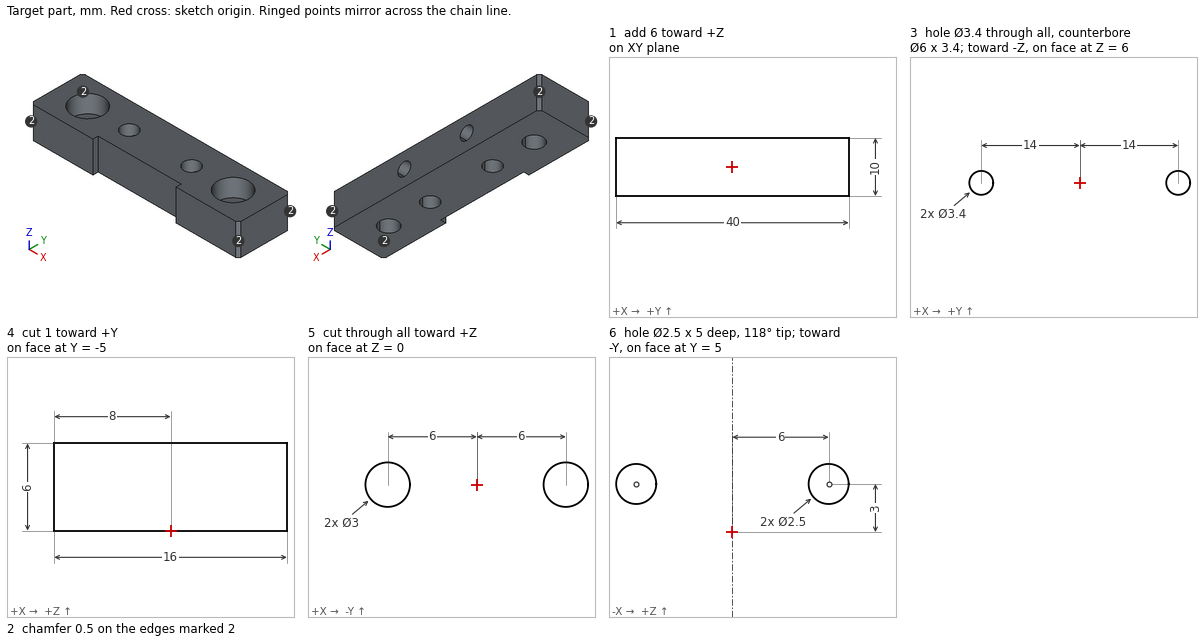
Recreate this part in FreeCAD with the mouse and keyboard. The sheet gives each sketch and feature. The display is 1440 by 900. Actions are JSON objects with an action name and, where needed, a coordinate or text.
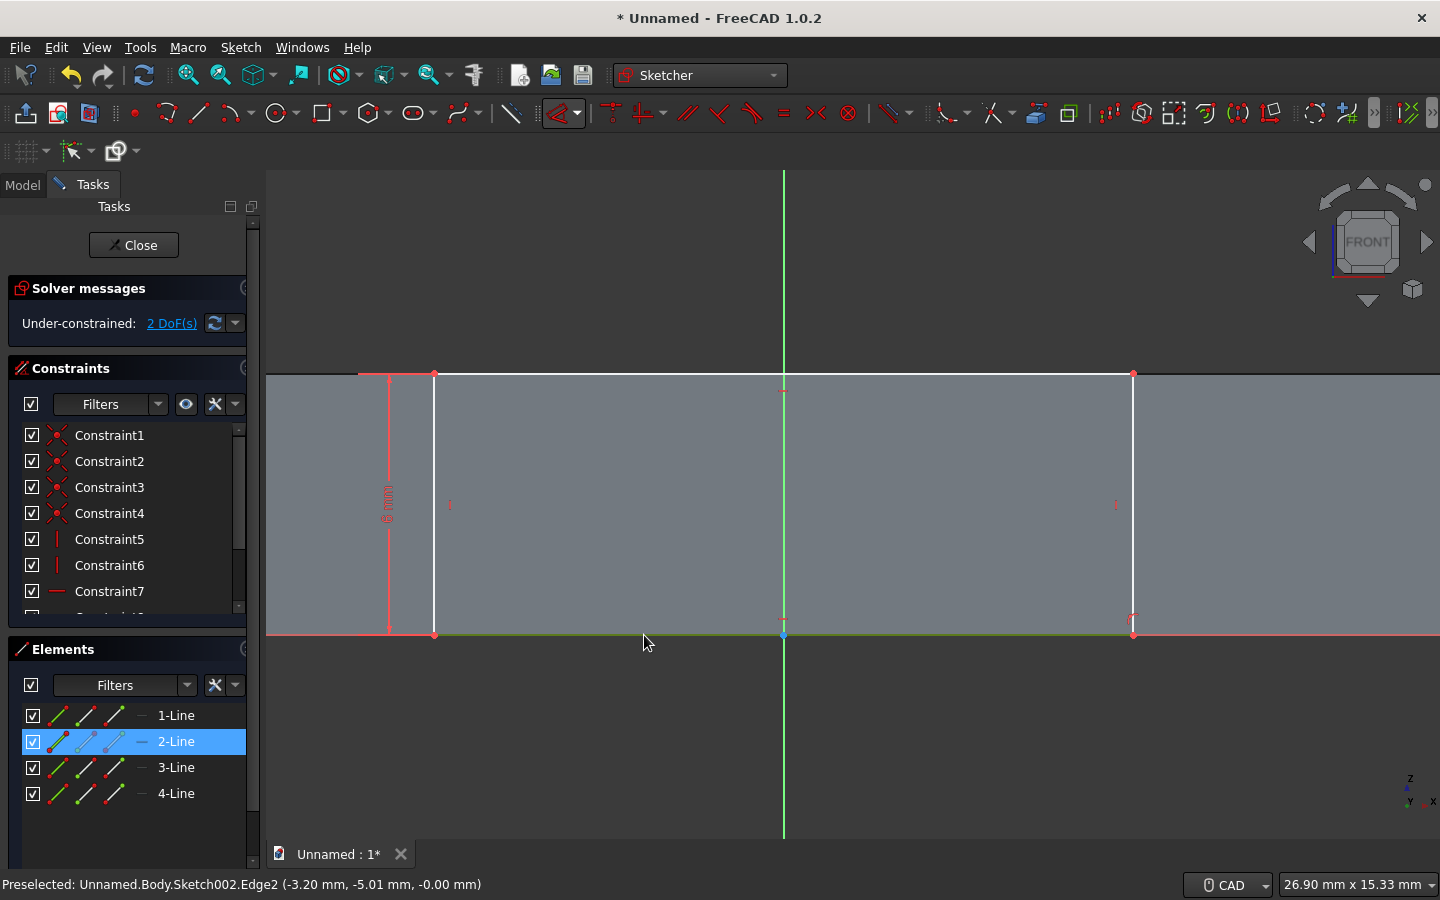
{"action": "left_click", "coordinate": [580, 114]}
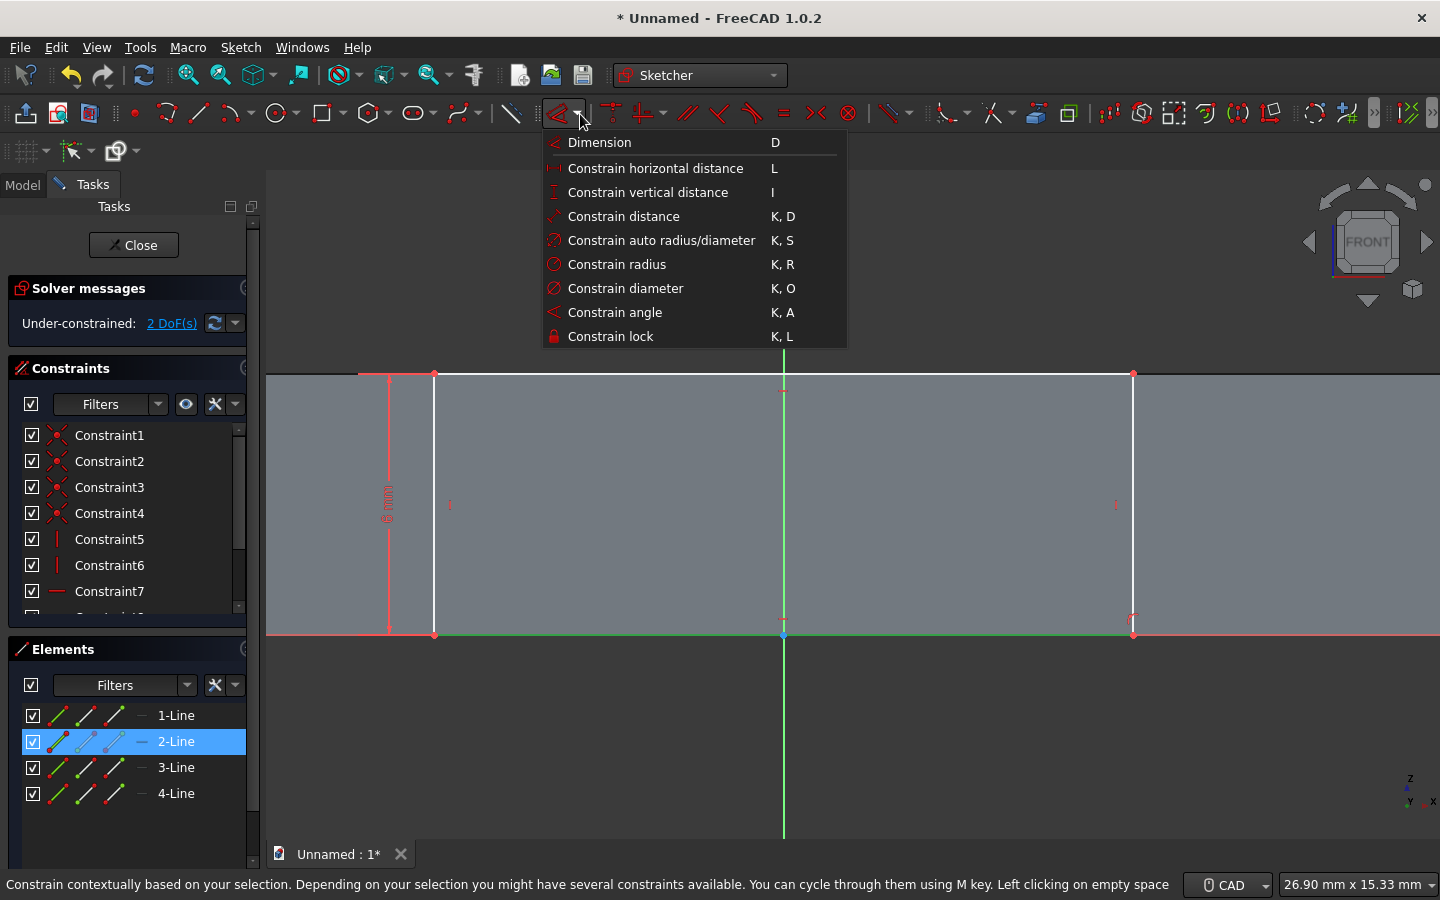
{"action": "left_click", "coordinate": [695, 168]}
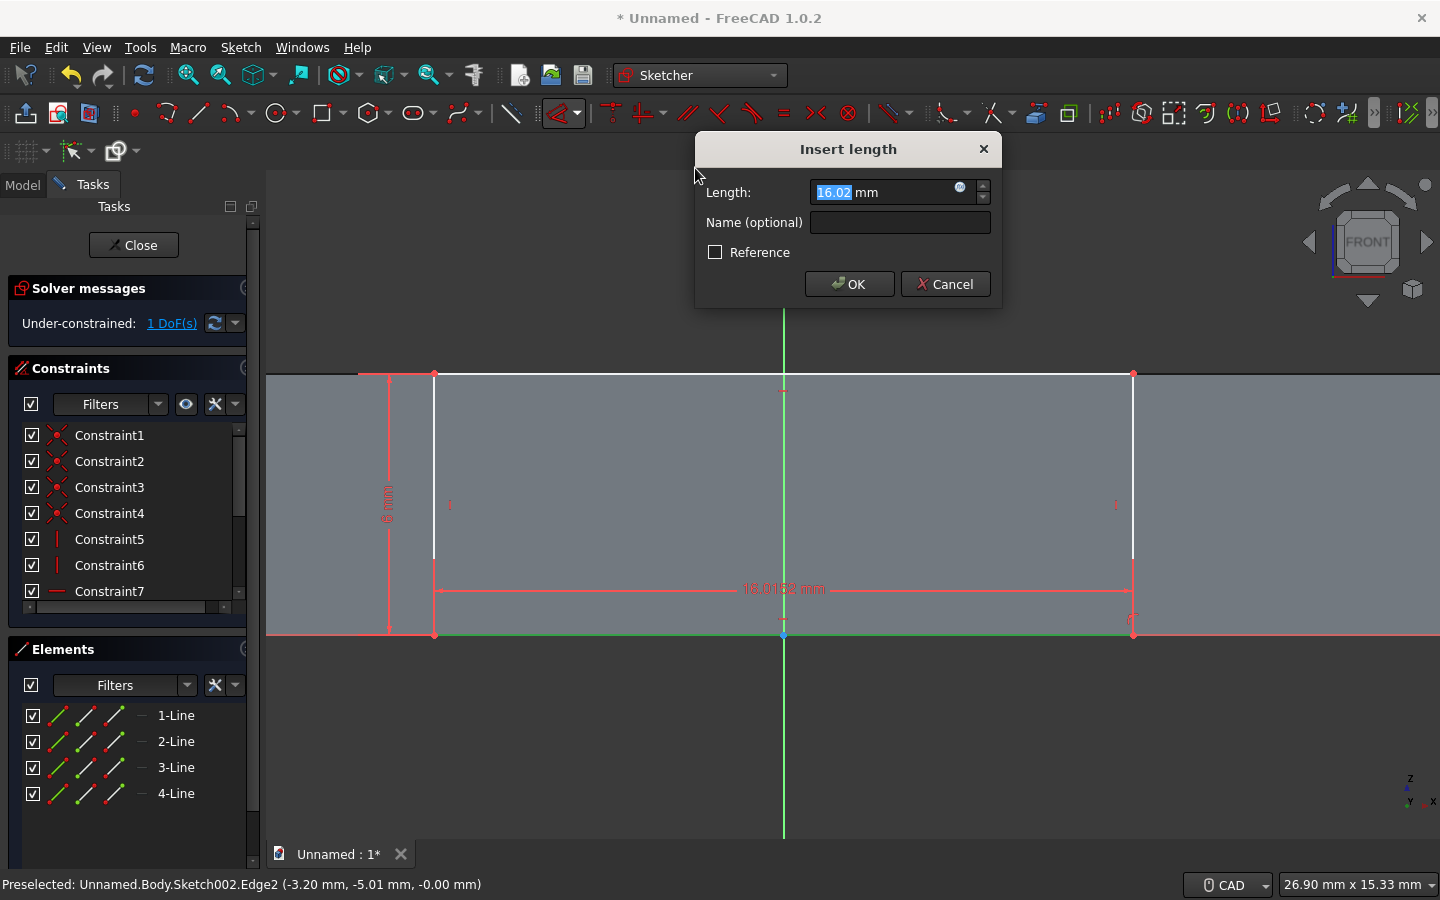
{"action": "type", "text": "16"}
{"action": "key", "text": "Return"}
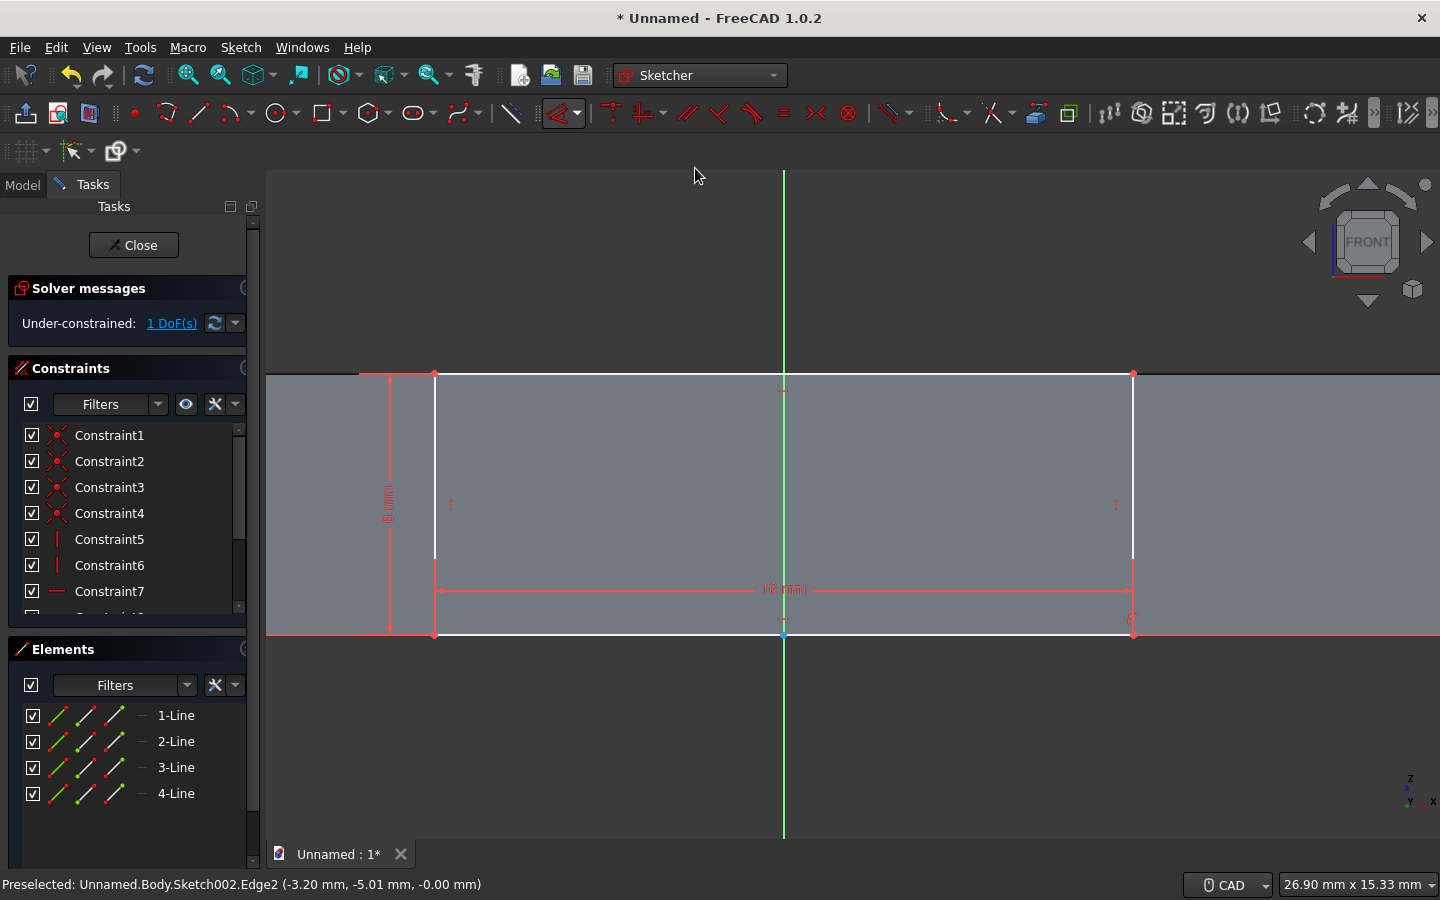
{"action": "left_click", "coordinate": [435, 374]}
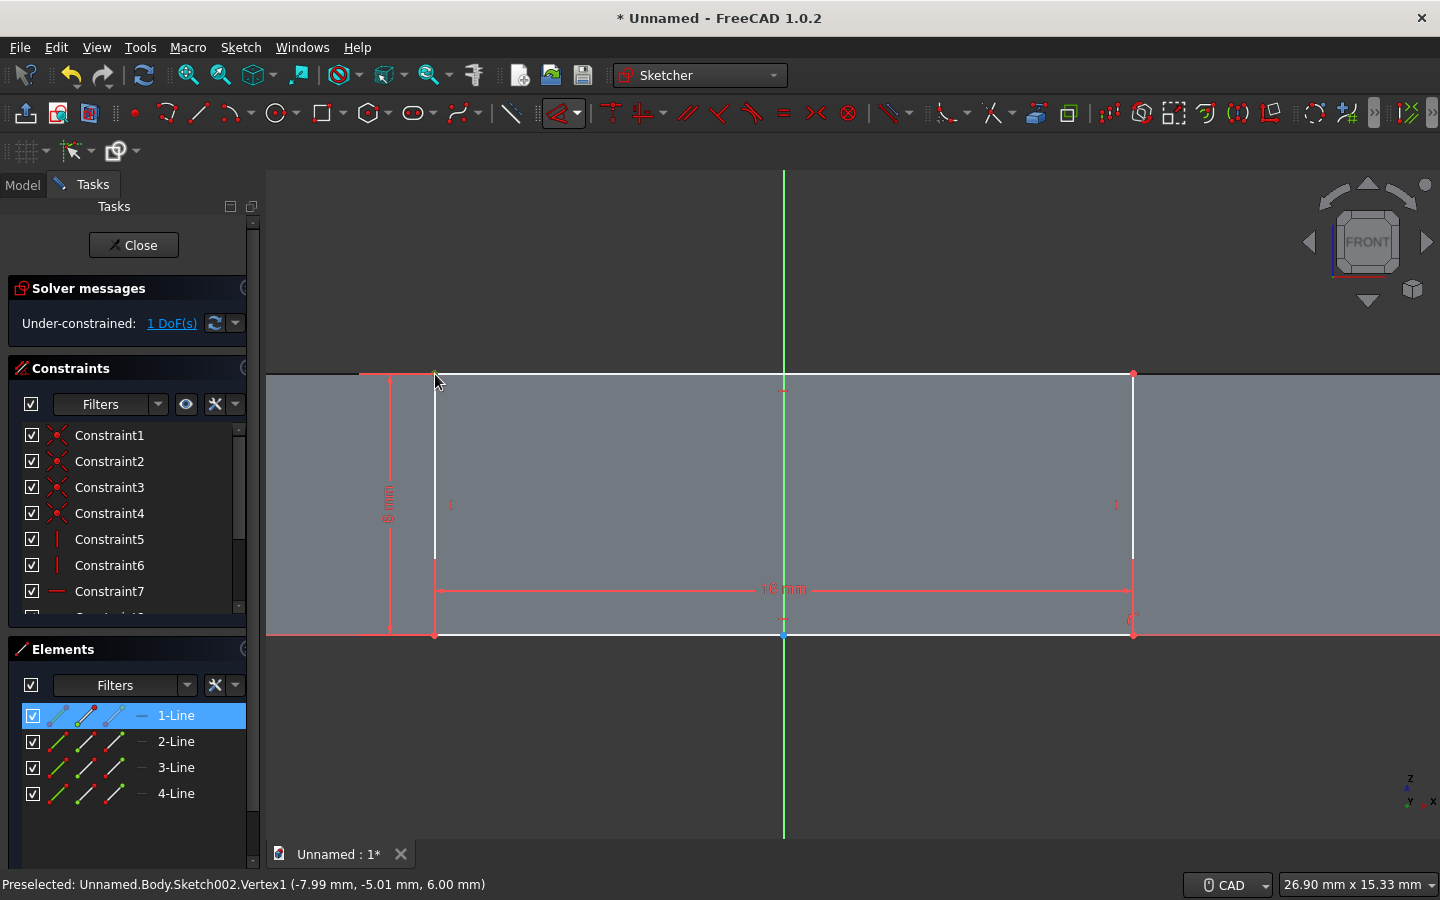
{"action": "key", "text": "l"}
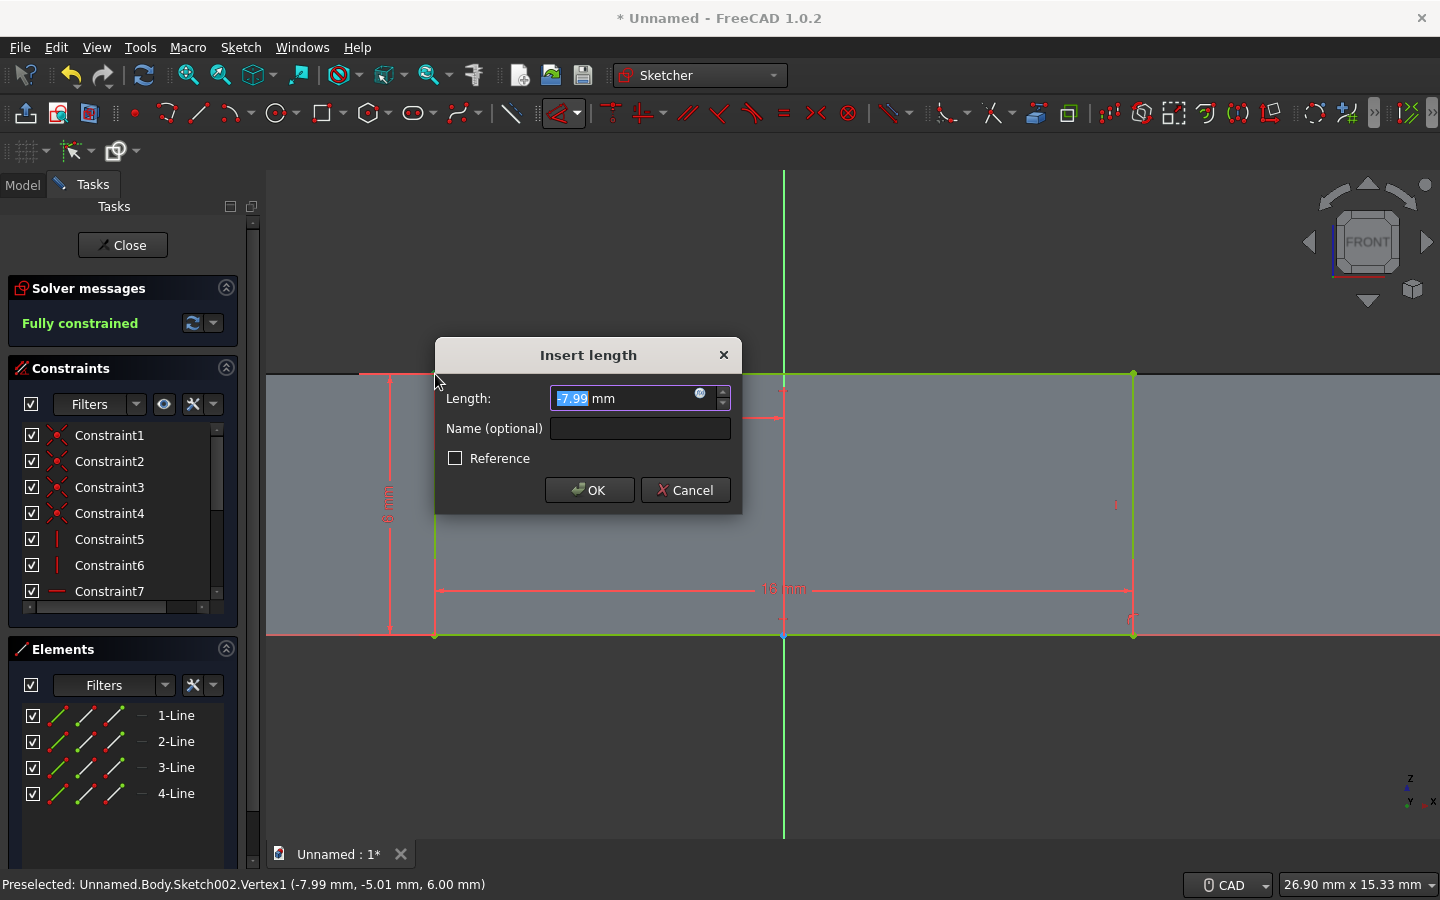
{"action": "type", "text": "-8"}
{"action": "key", "text": "Return"}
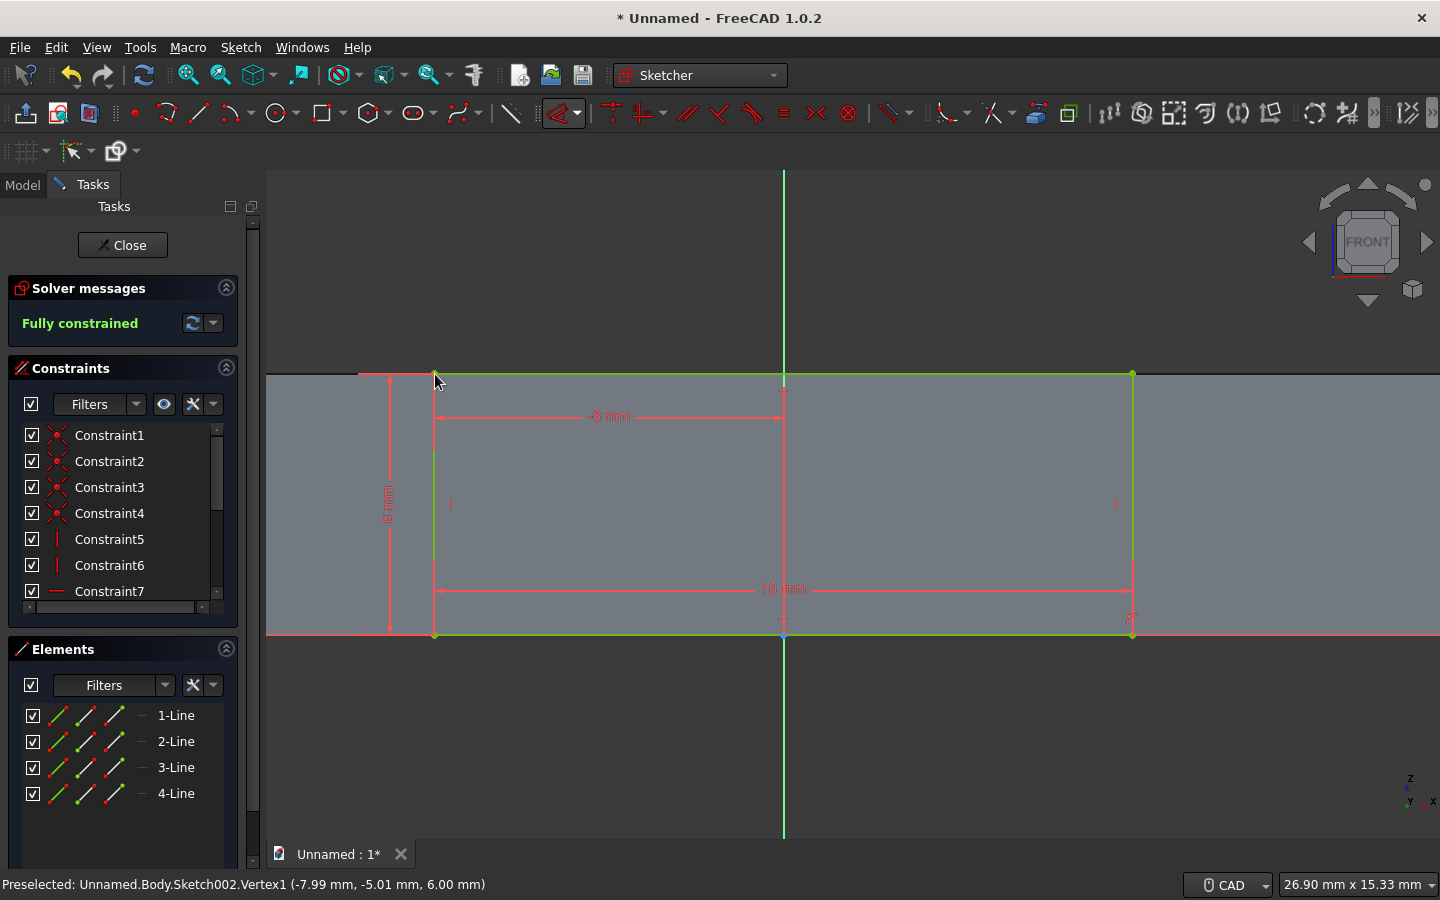
{"action": "left_click", "coordinate": [123, 245]}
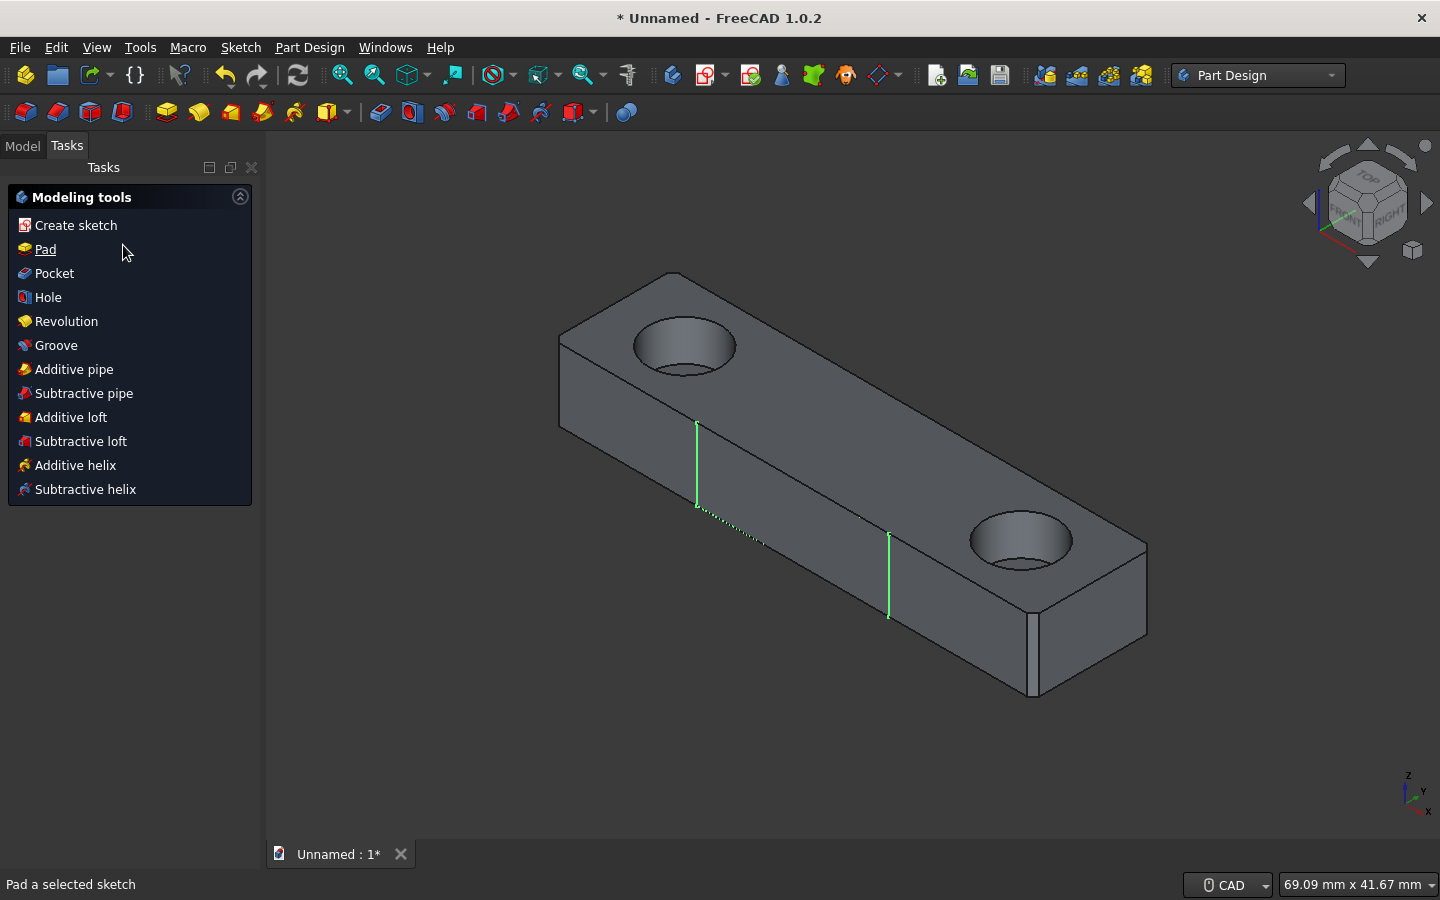
{"action": "left_click", "coordinate": [382, 112]}